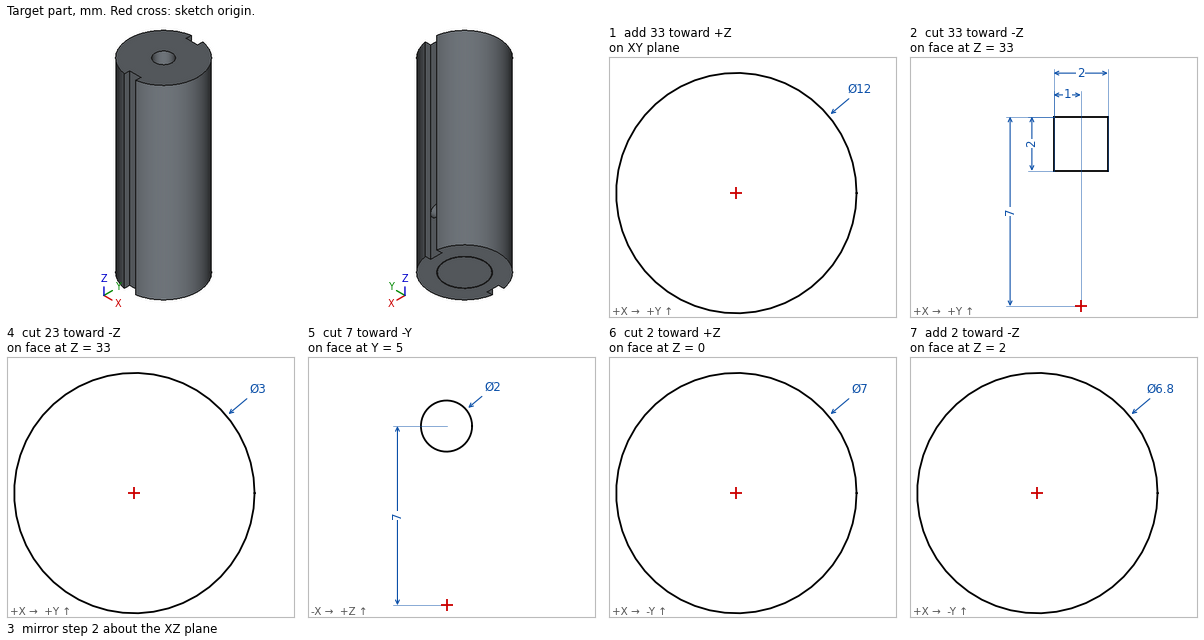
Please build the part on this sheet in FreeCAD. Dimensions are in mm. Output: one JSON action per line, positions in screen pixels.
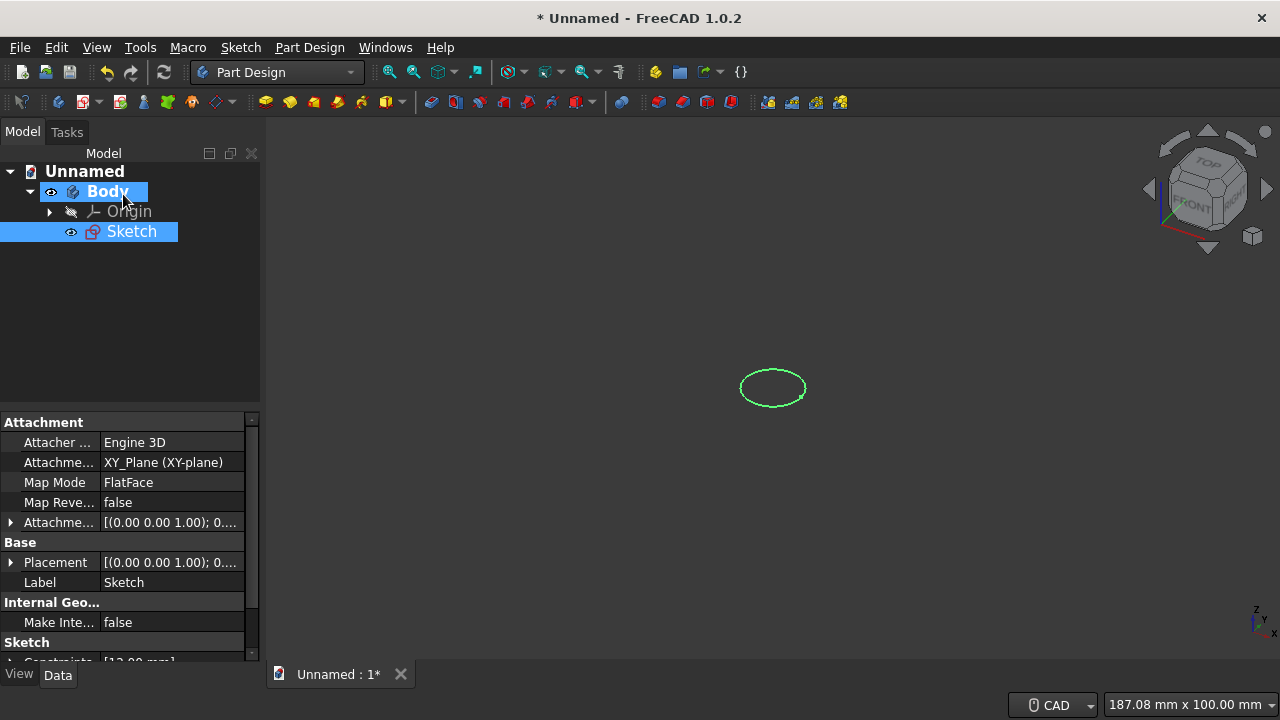
{"action": "left_click", "coordinate": [266, 102]}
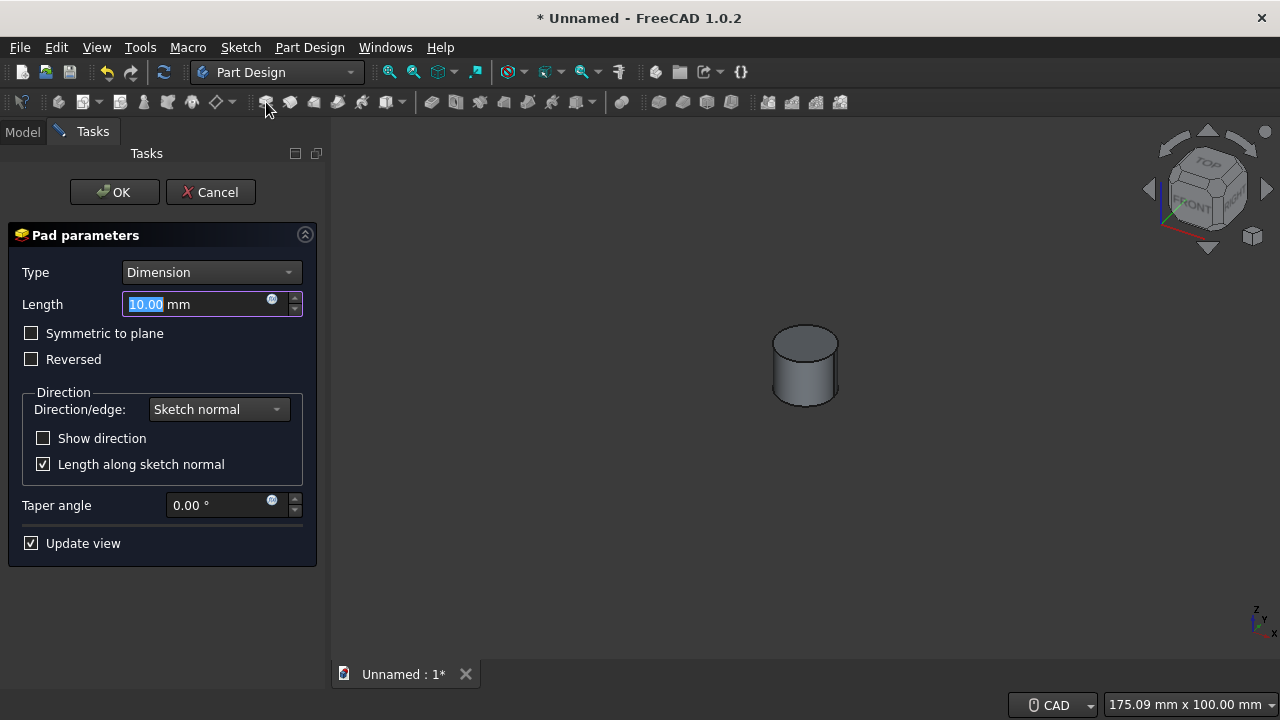
{"action": "type", "text": "33"}
{"action": "key", "text": "Tab"}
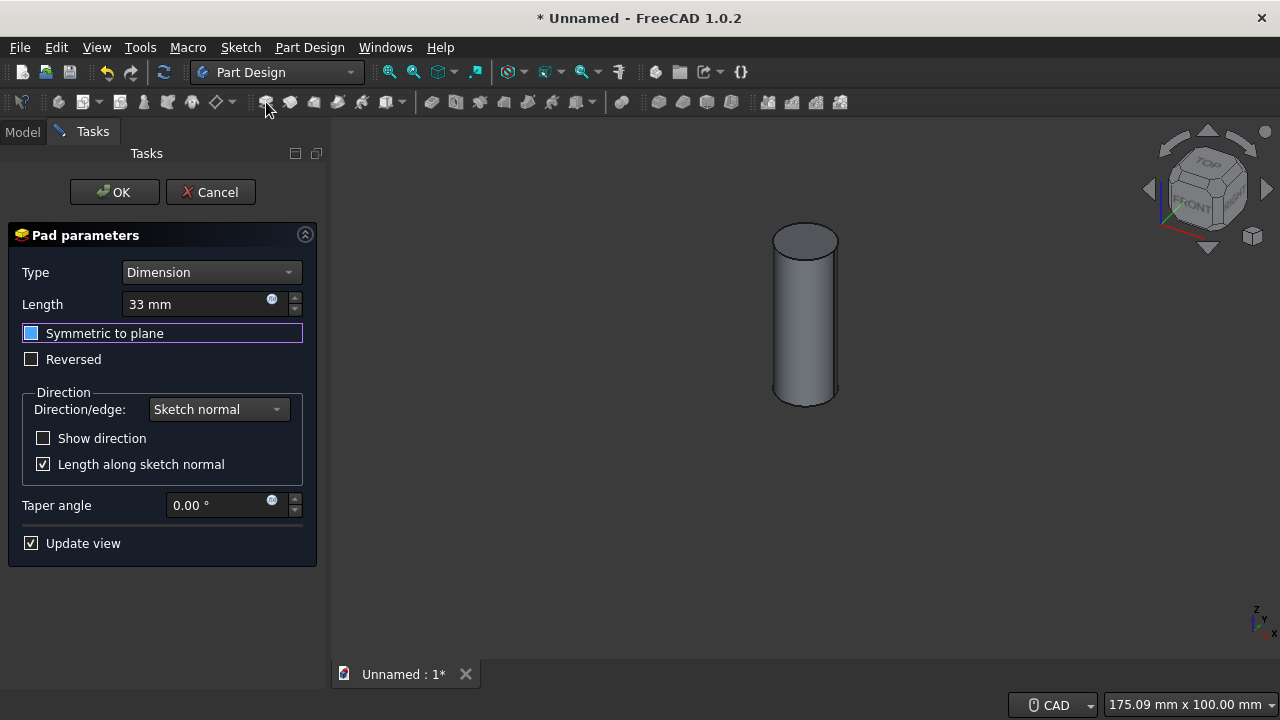
{"action": "left_click", "coordinate": [115, 192]}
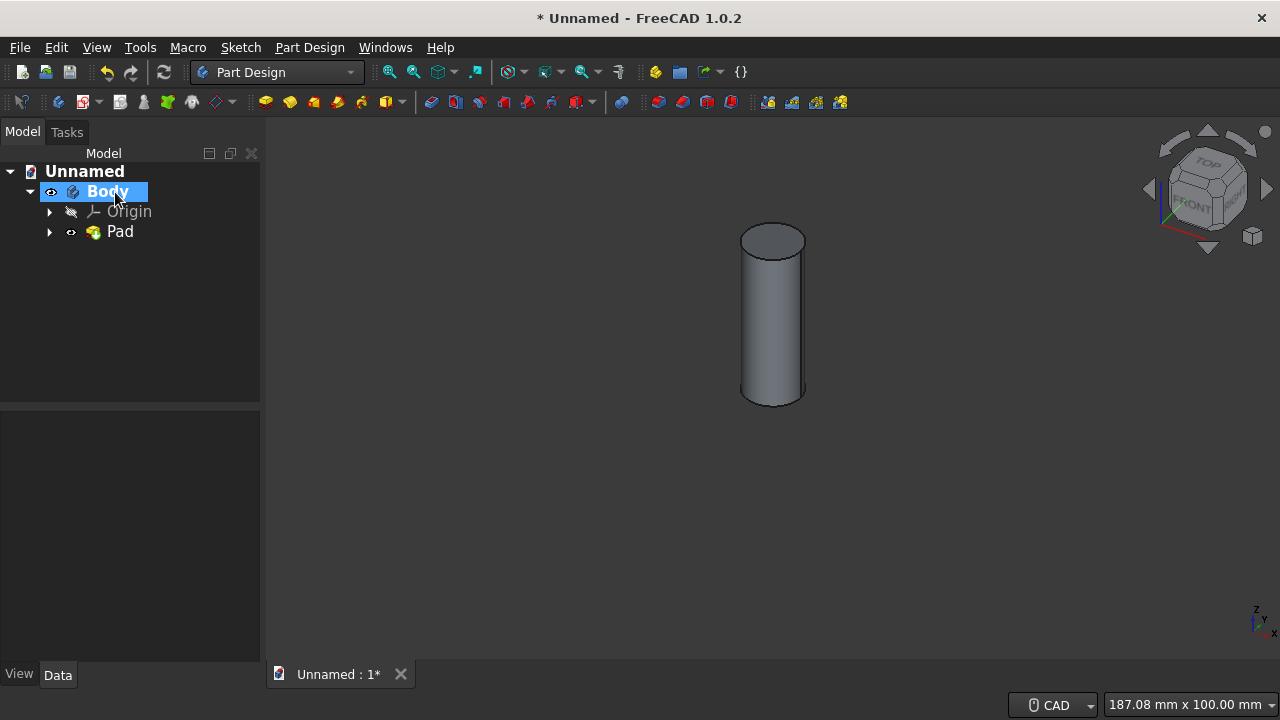
{"action": "key", "text": "v f"}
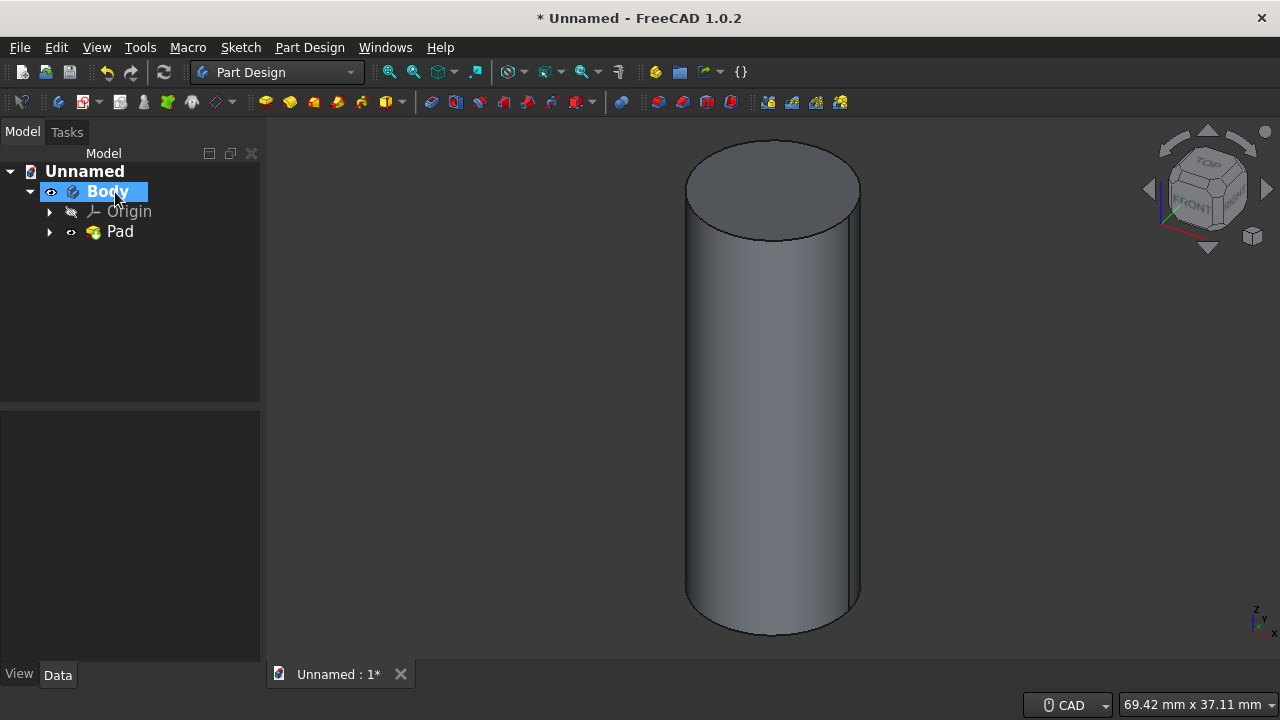
{"action": "left_click", "coordinate": [773, 190]}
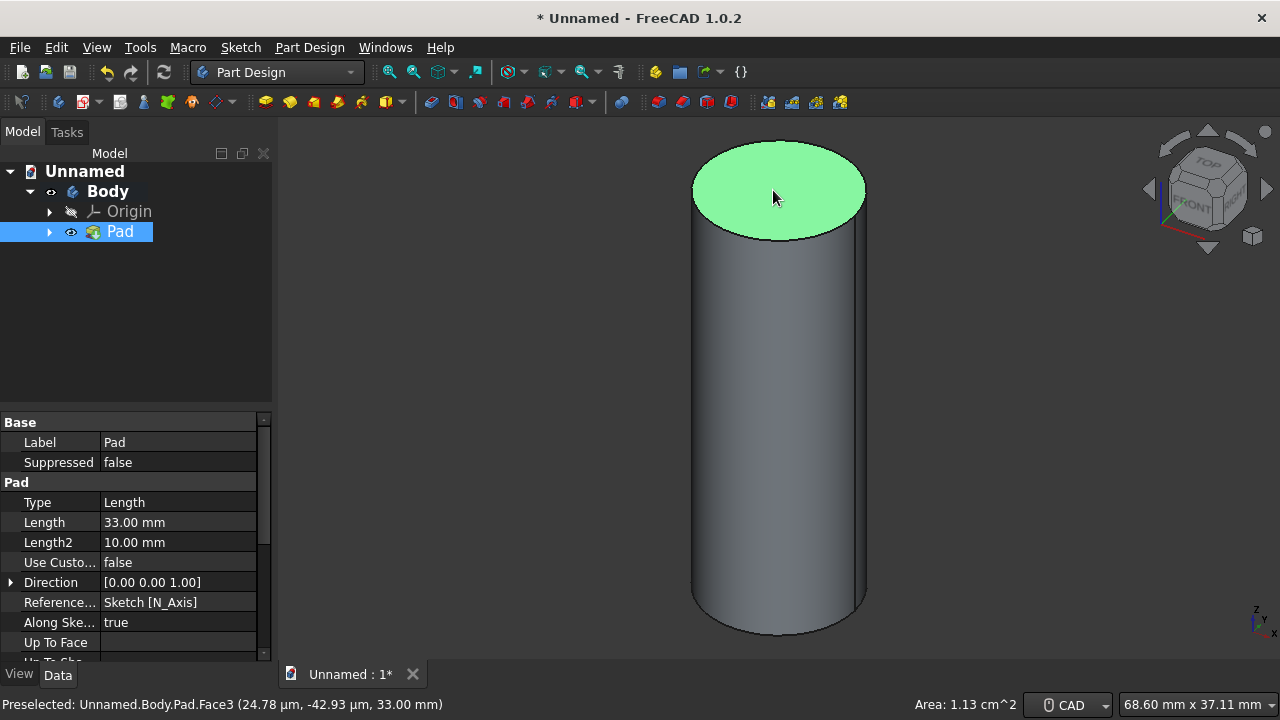
{"action": "left_click", "coordinate": [84, 102]}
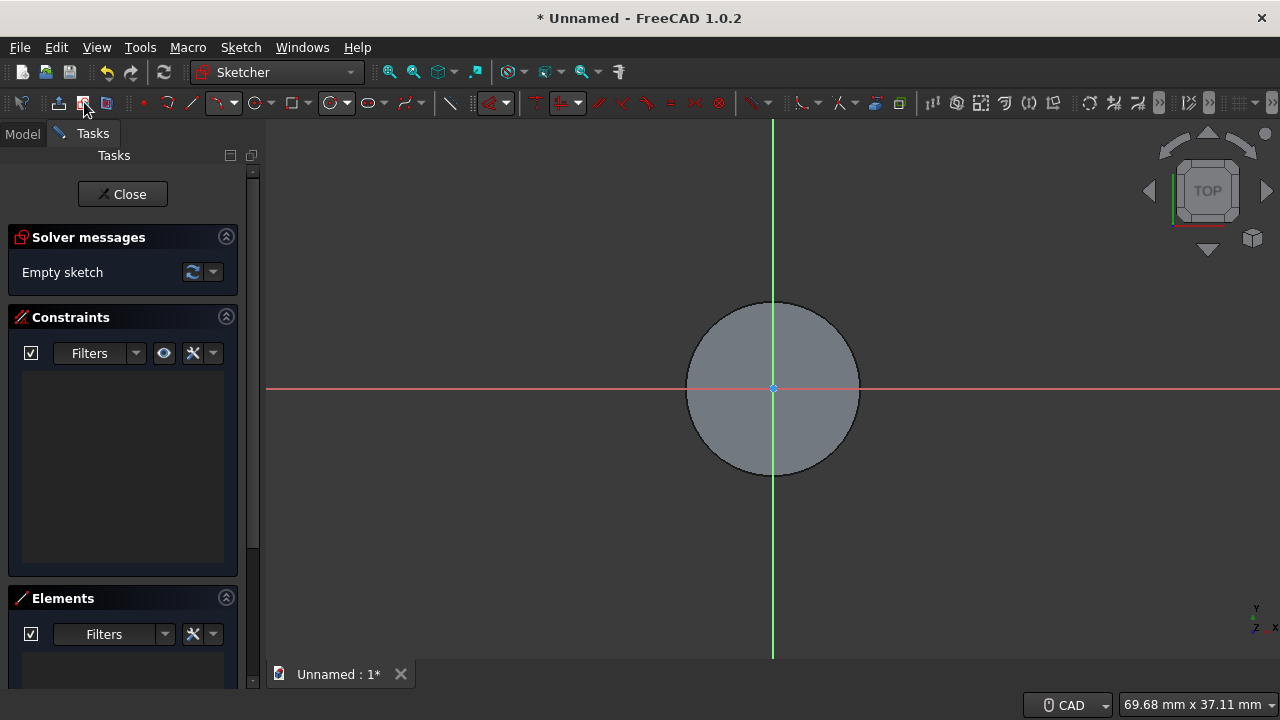
{"action": "scroll", "coordinate": [780, 293], "scroll_direction": "up", "scroll_amount": 12}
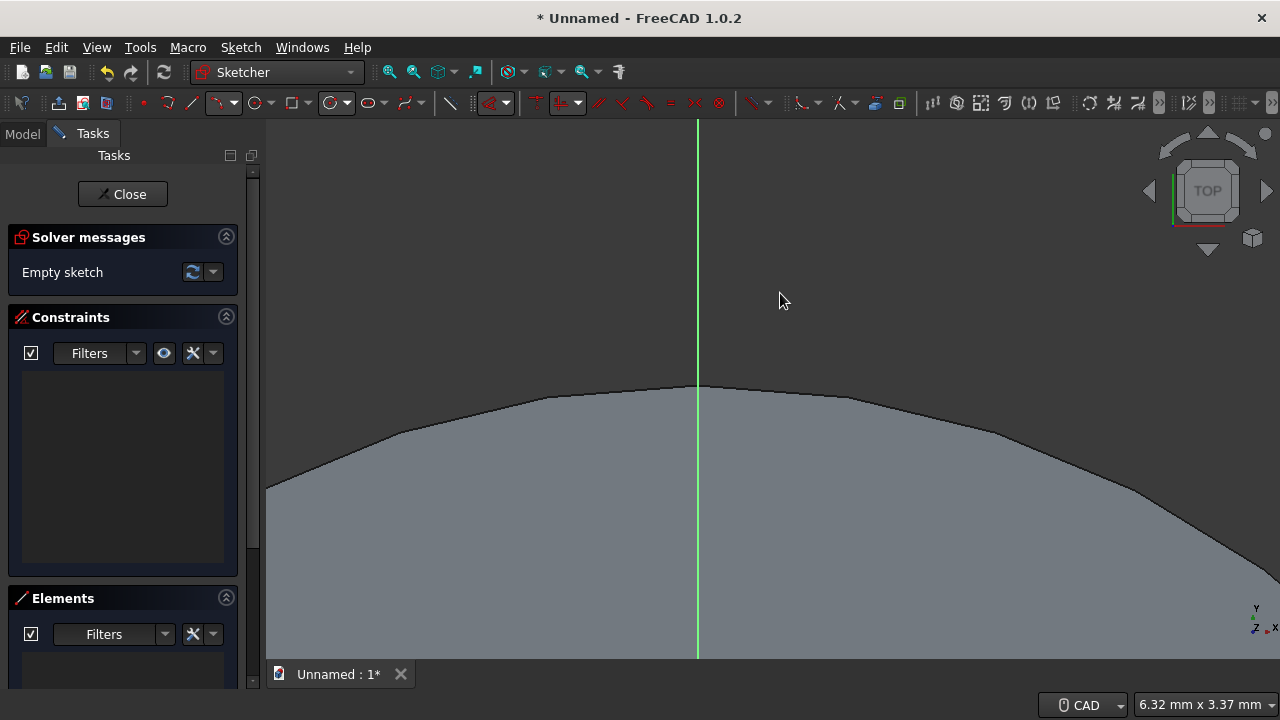
{"action": "key", "text": "g r"}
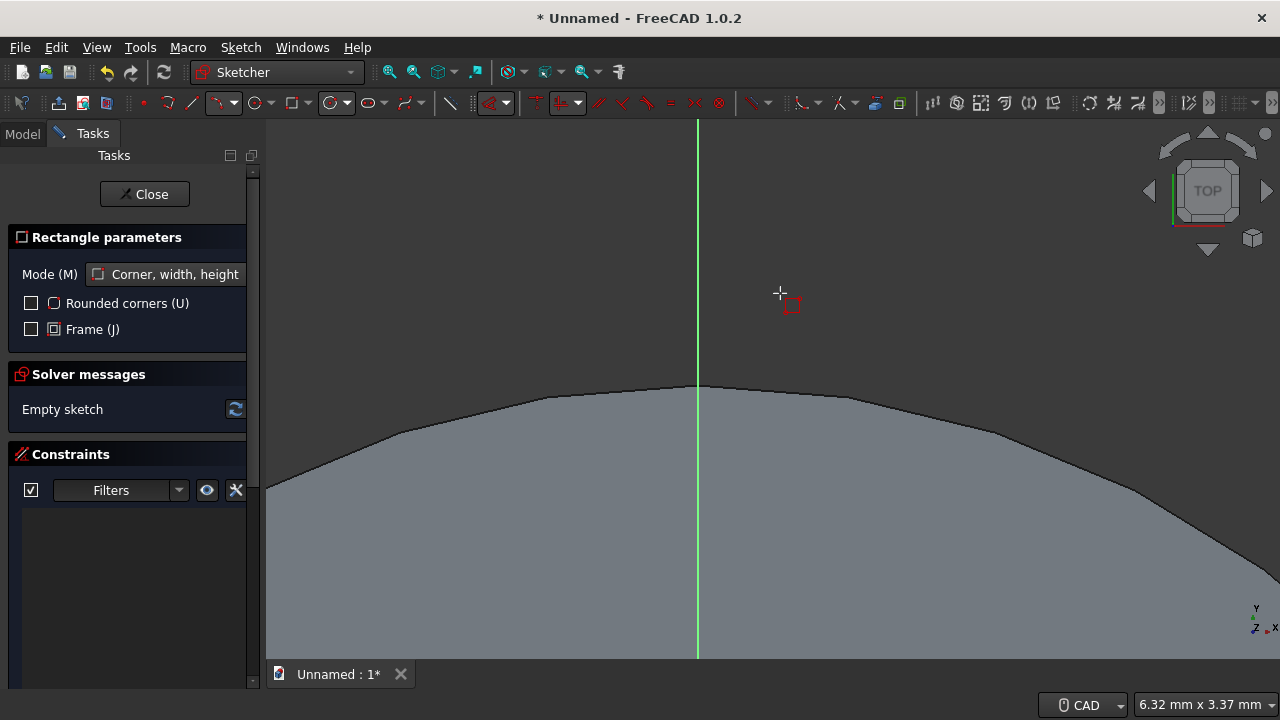
{"action": "left_click", "coordinate": [537, 225]}
{"action": "left_click", "coordinate": [858, 546]}
{"action": "key", "text": "Escape"}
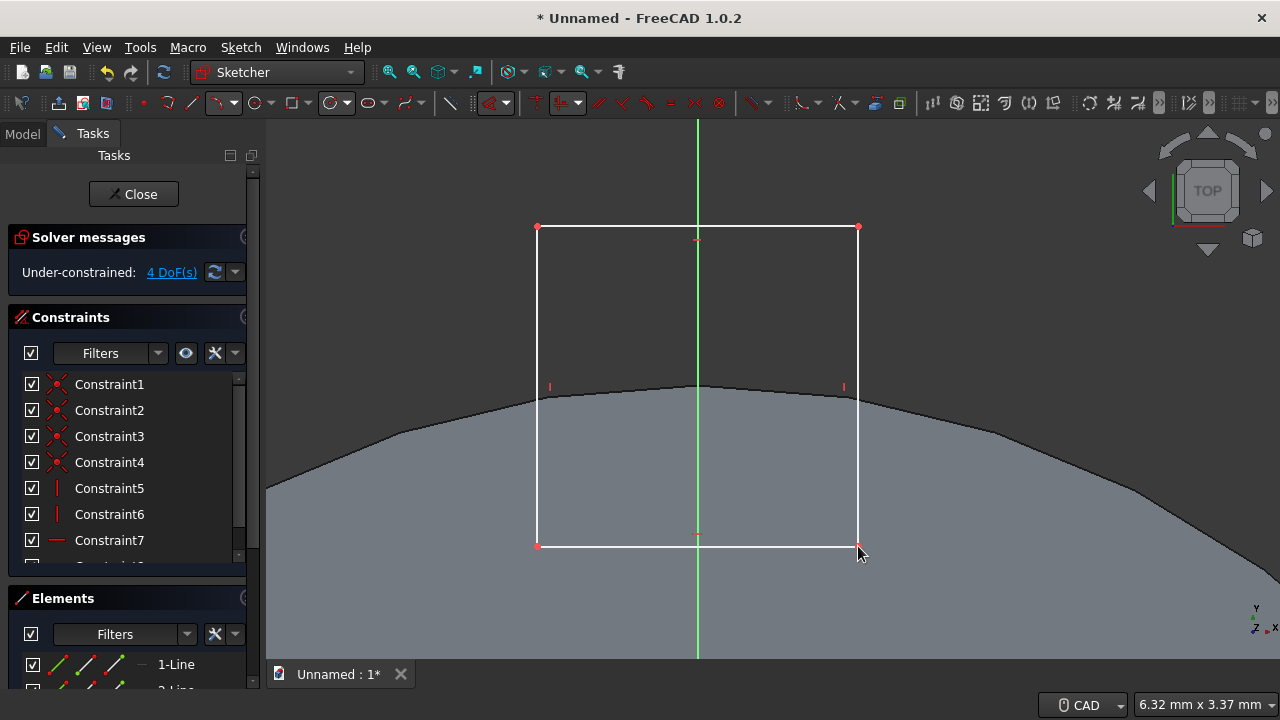
{"action": "key", "text": "d"}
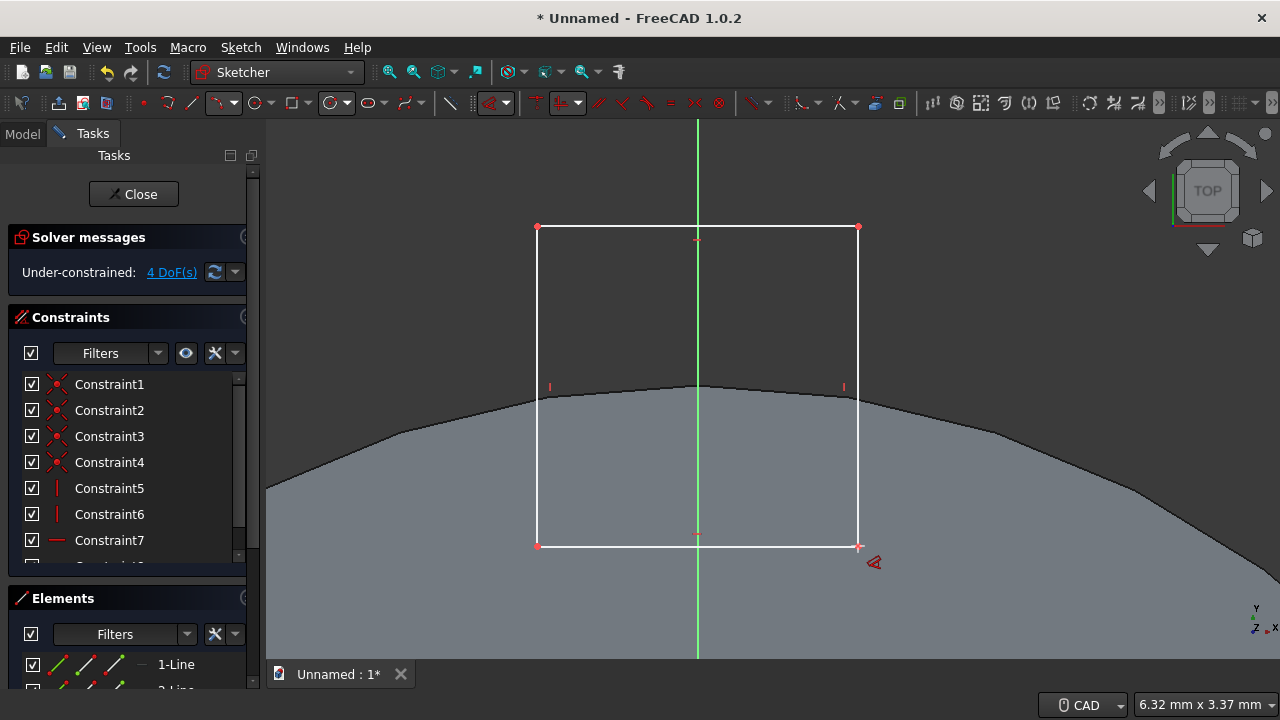
{"action": "left_click", "coordinate": [537, 322]}
{"action": "left_click", "coordinate": [503, 387]}